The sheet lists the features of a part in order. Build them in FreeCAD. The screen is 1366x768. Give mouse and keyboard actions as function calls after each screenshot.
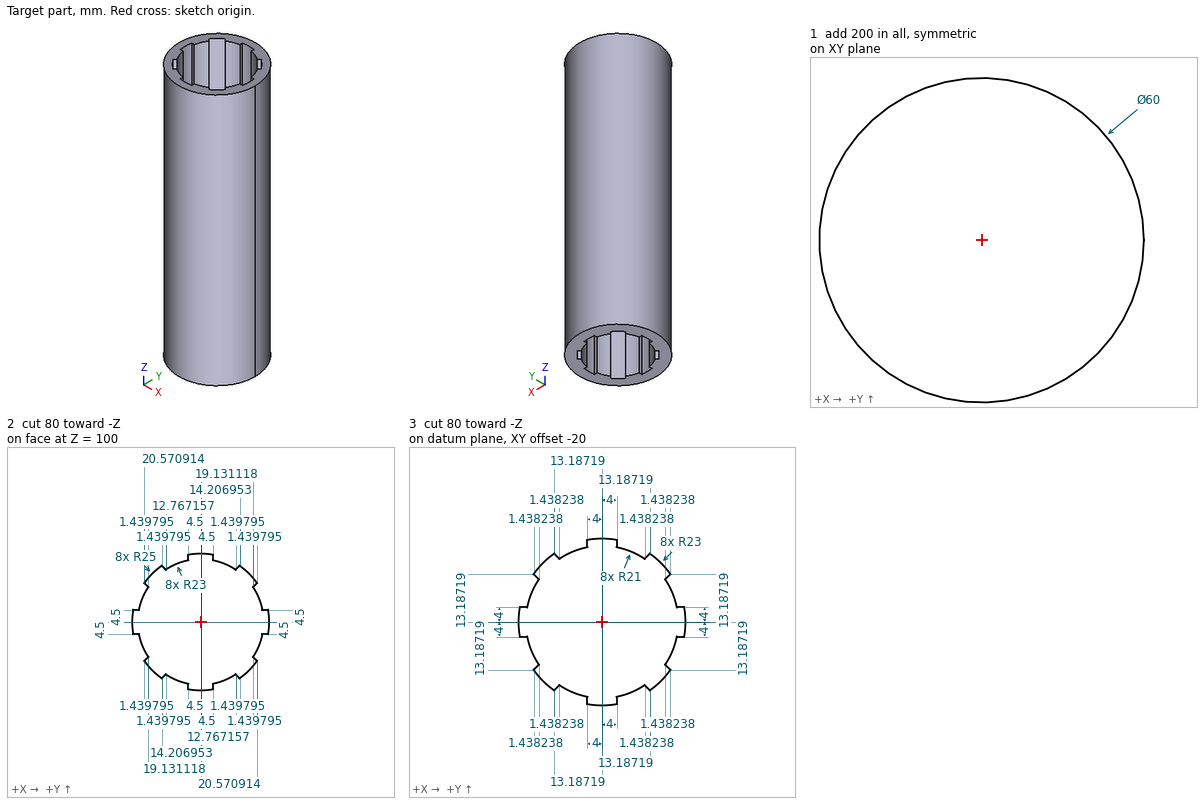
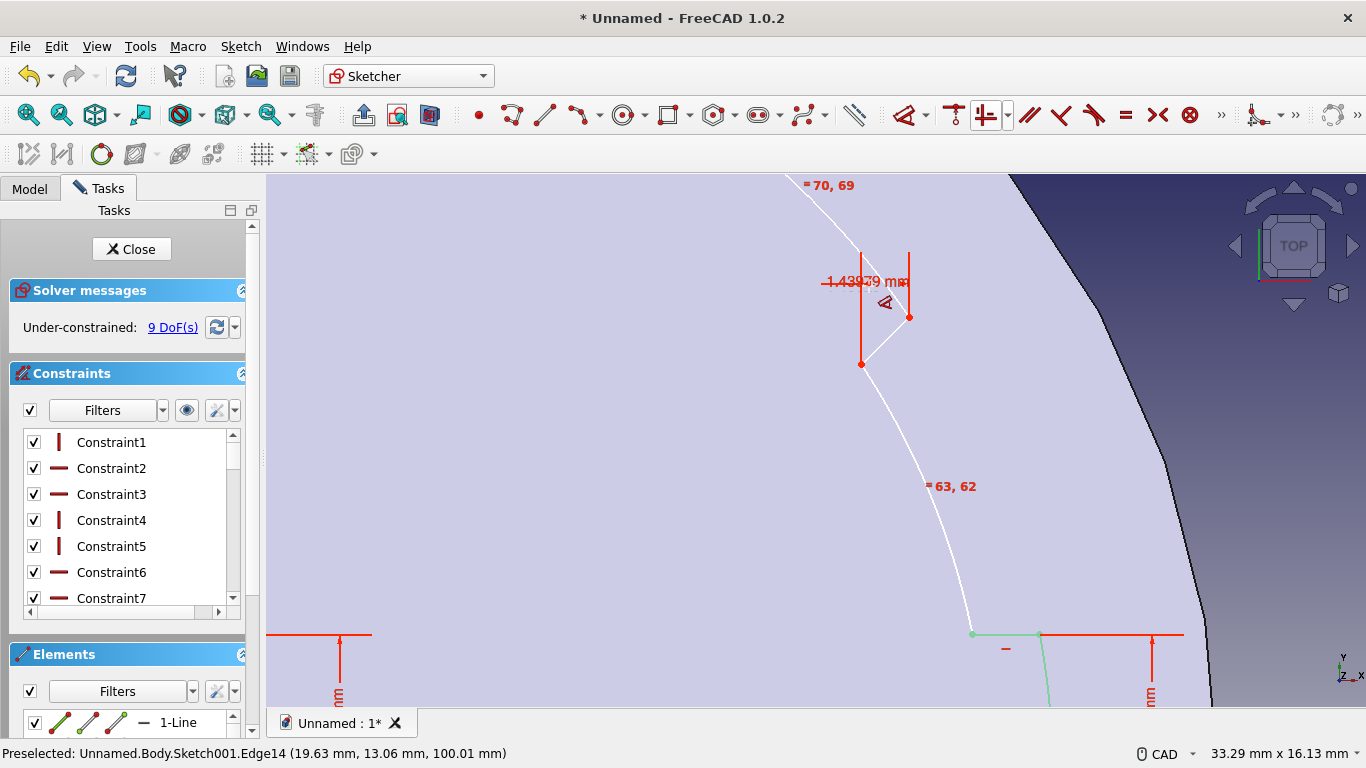
scroll(879, 354, down, 8)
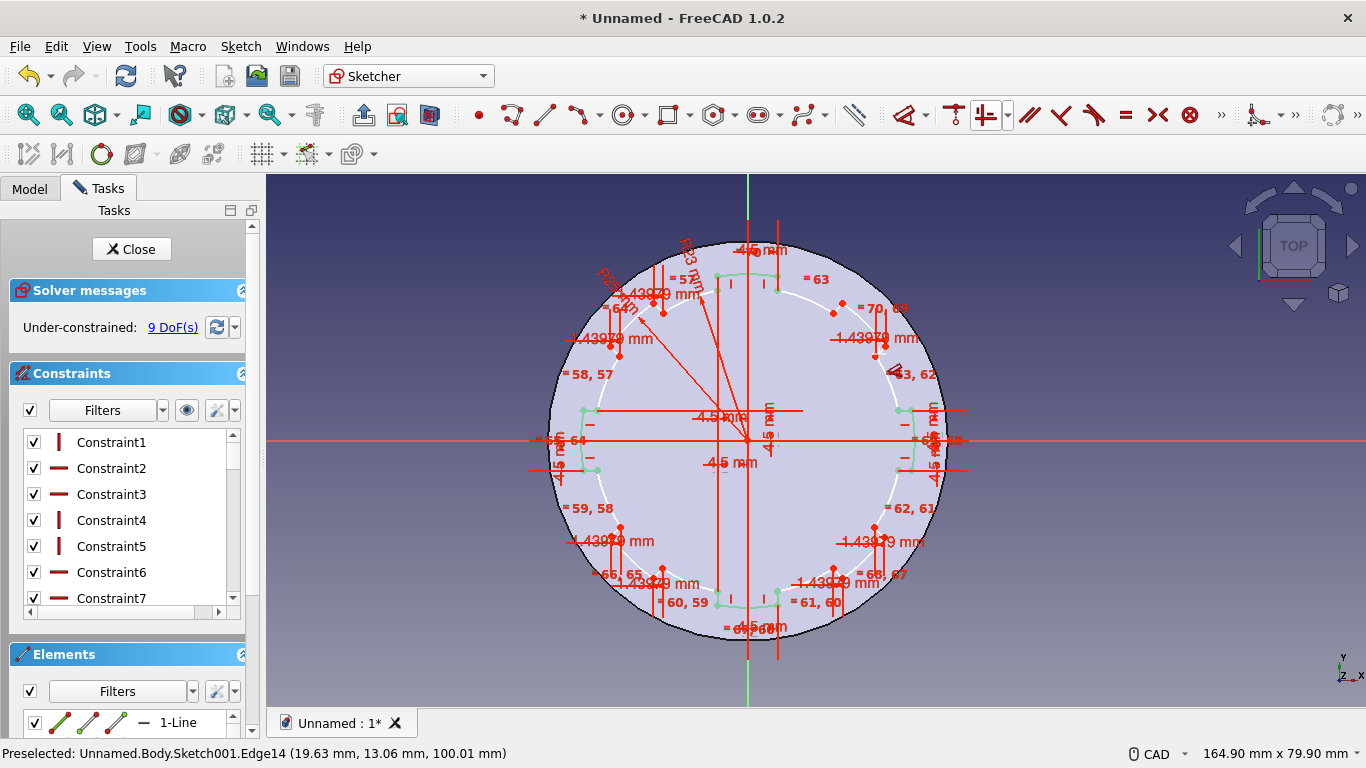
scroll(840, 307, up, 8)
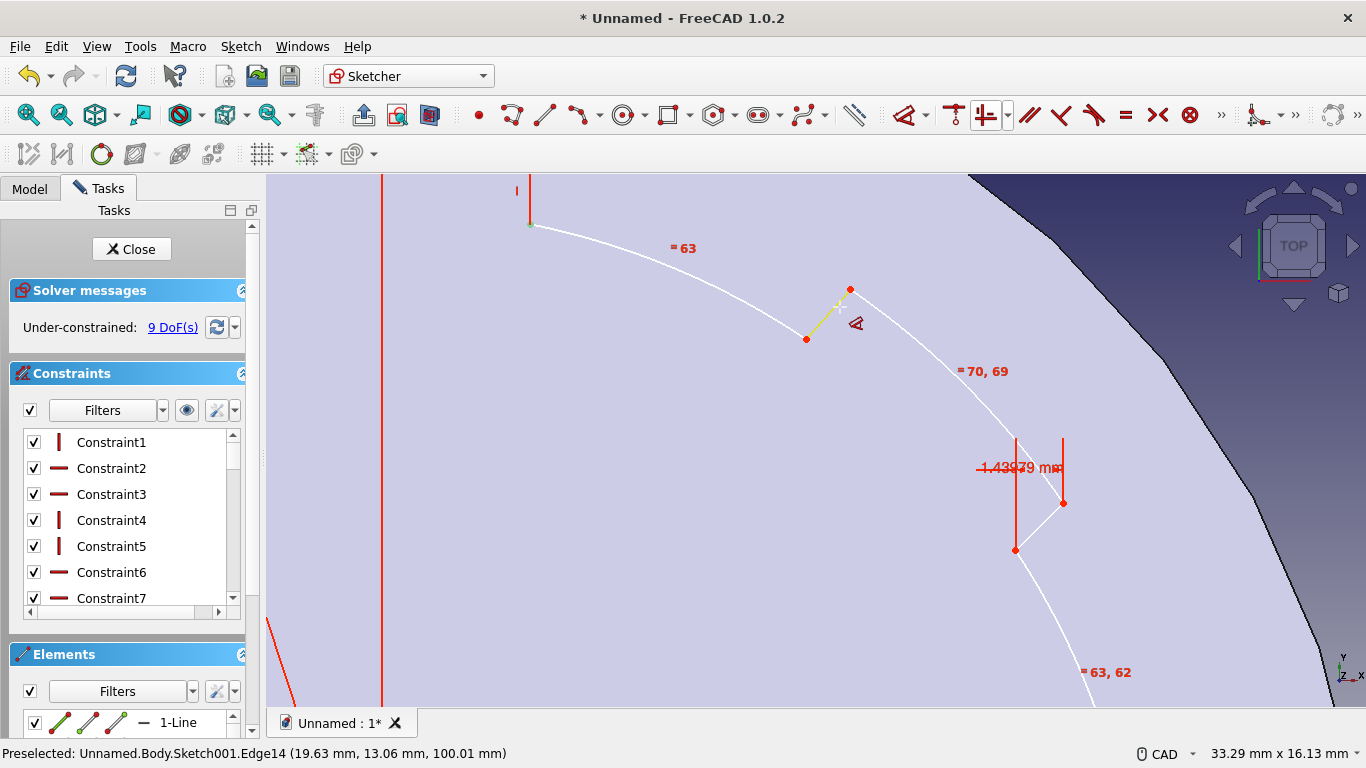
click(837, 305)
click(828, 256)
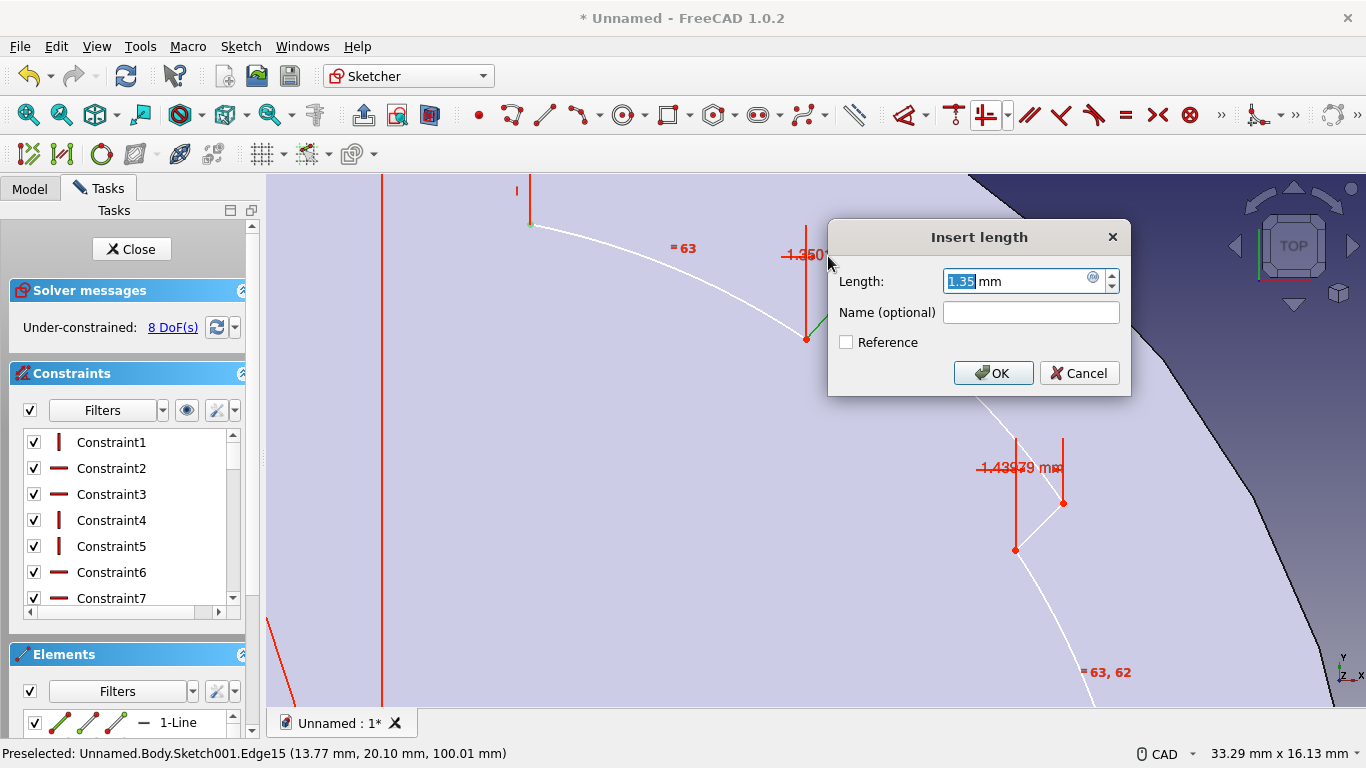
text(1.439795)
key(Return)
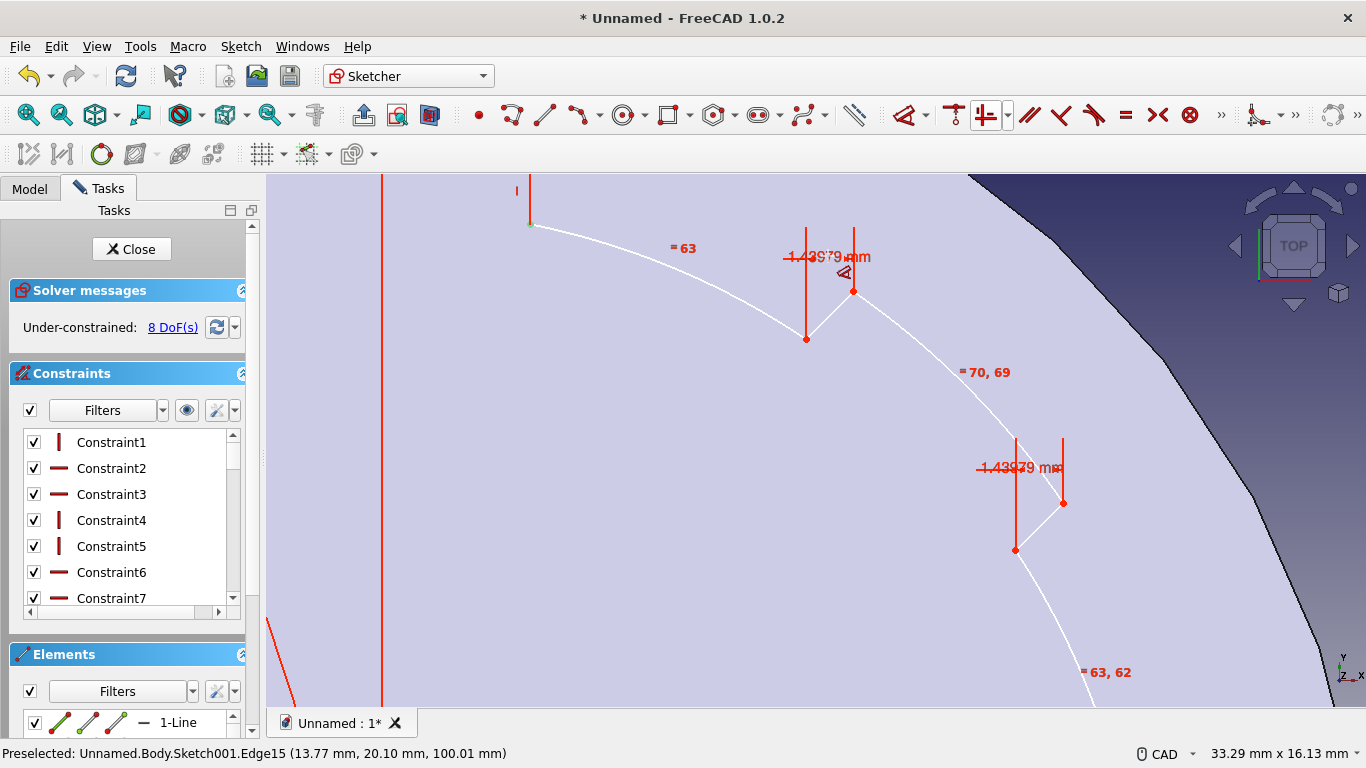
scroll(840, 307, down, 8)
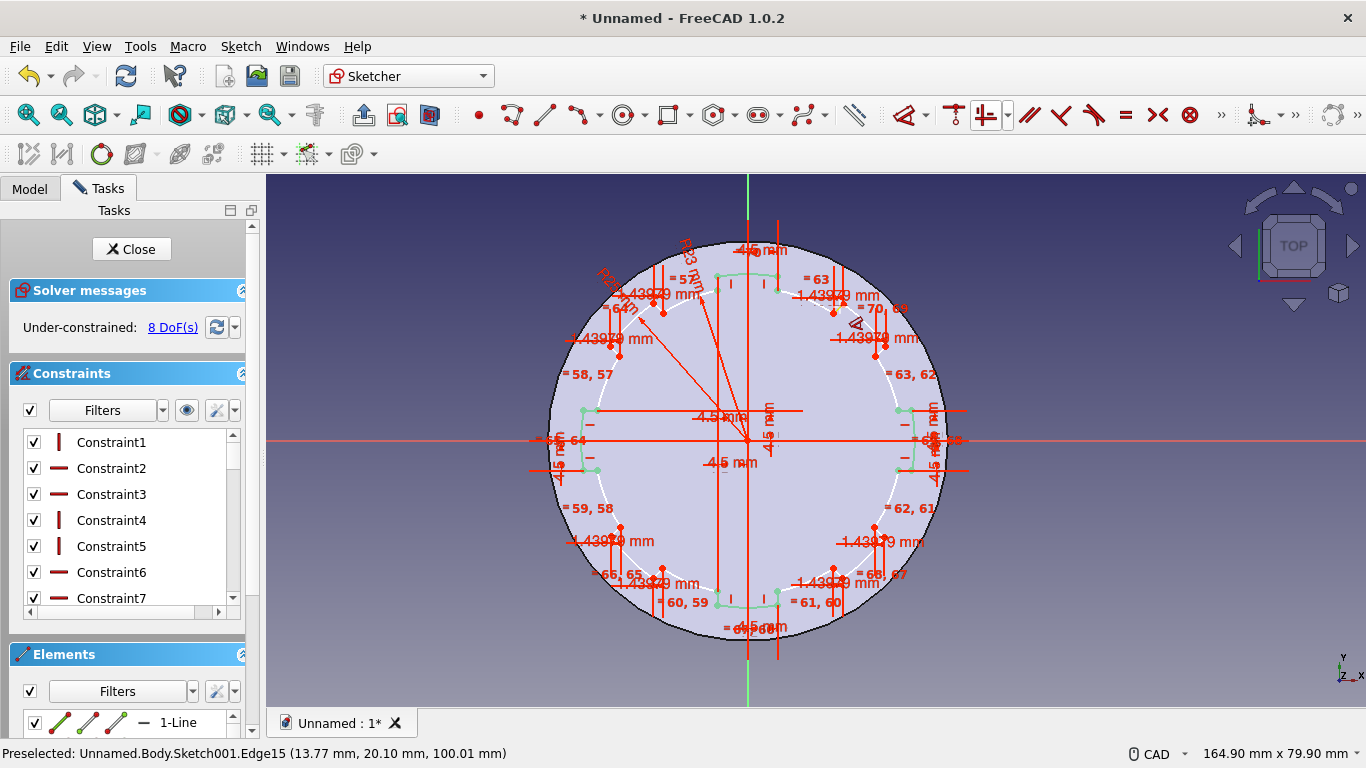
click(663, 313)
click(706, 499)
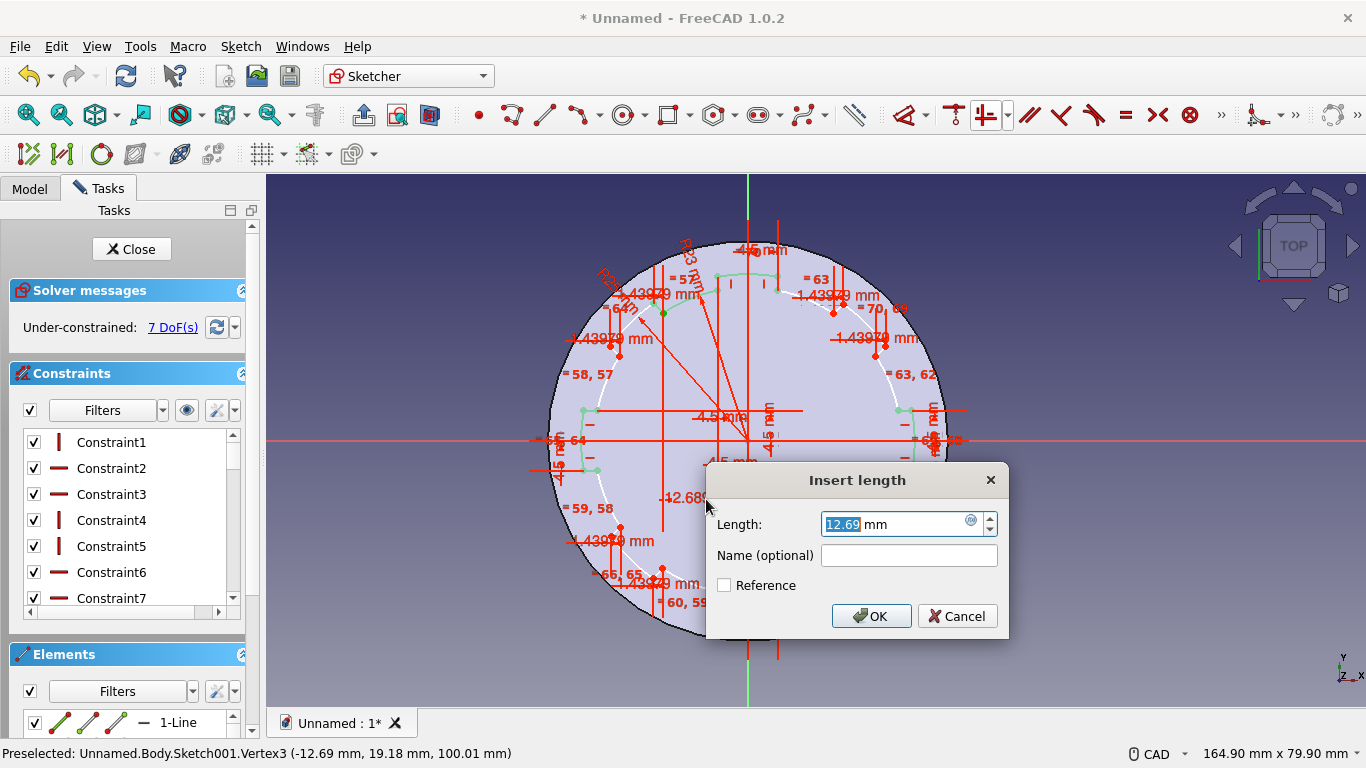
text(12.767157)
key(Return)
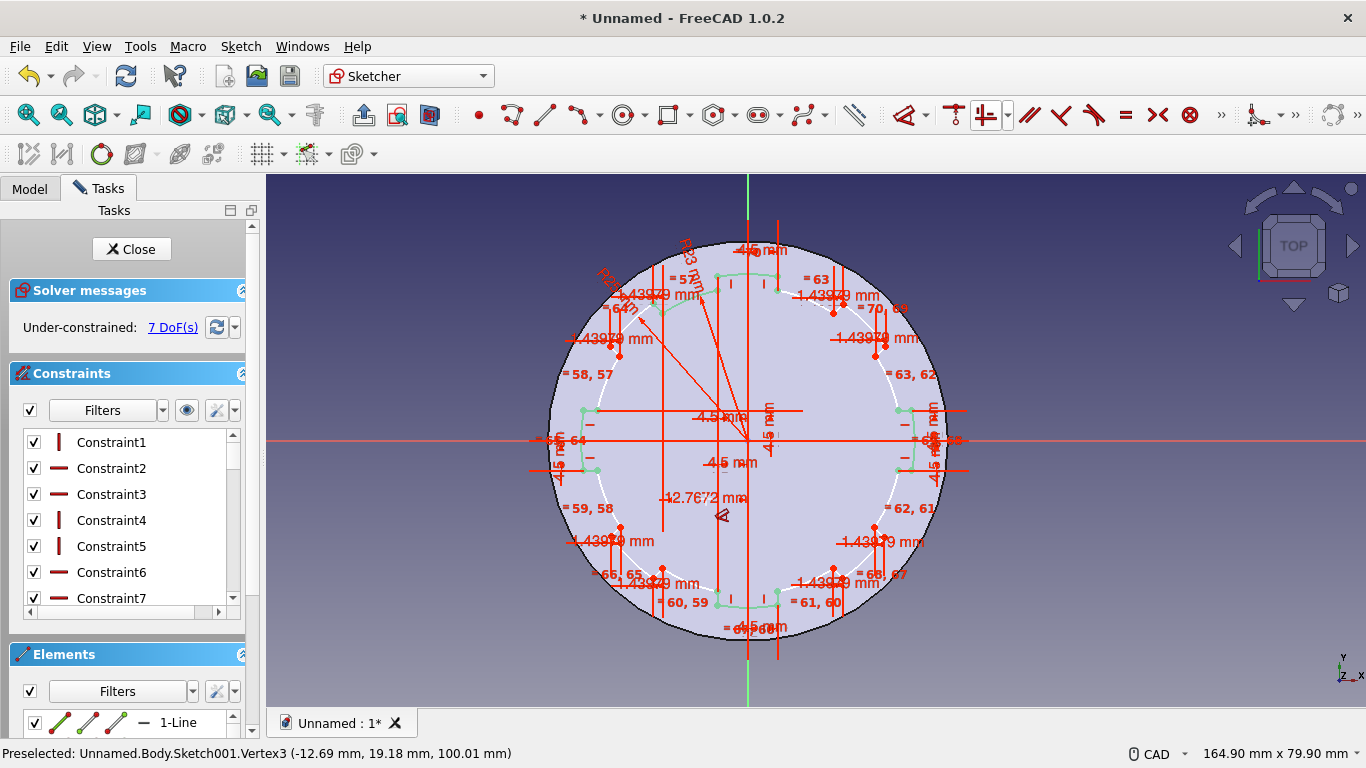
click(610, 347)
click(647, 475)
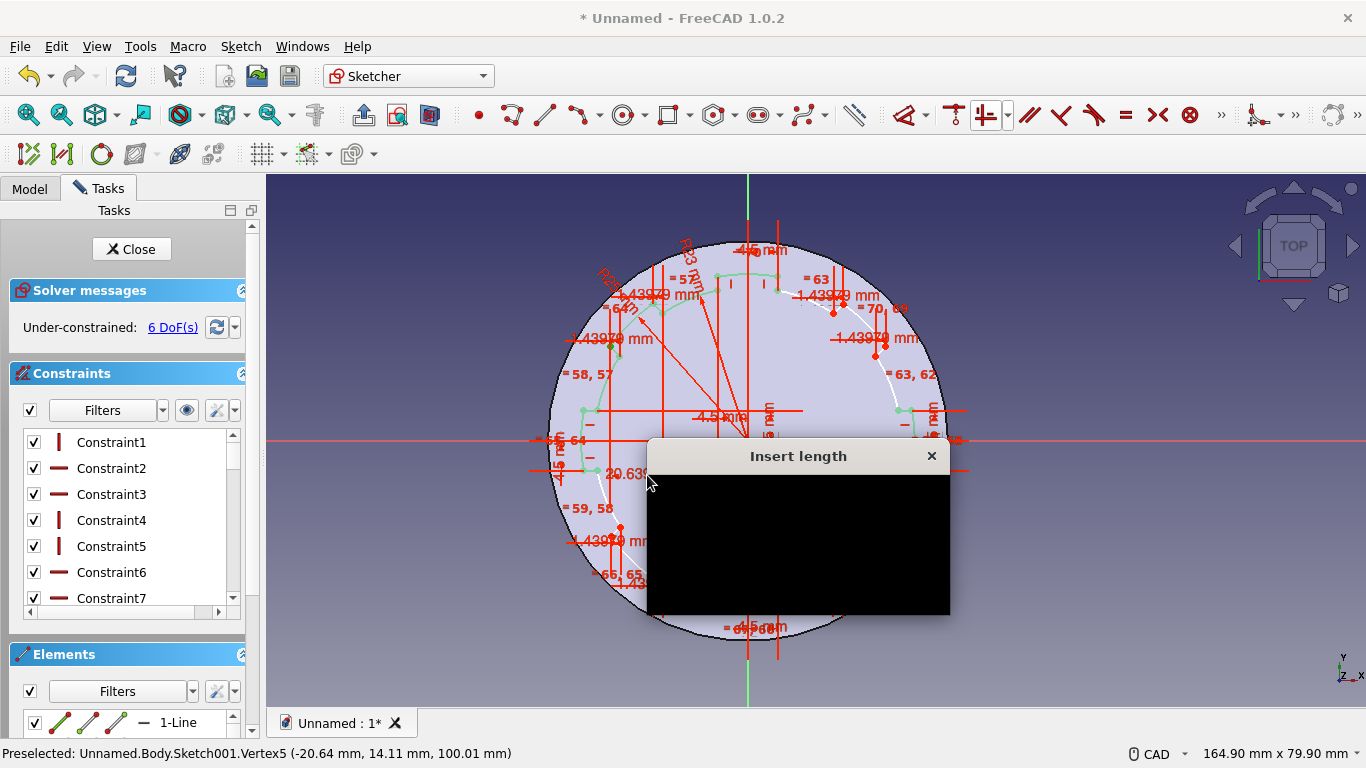
text(20.570914)
key(Return)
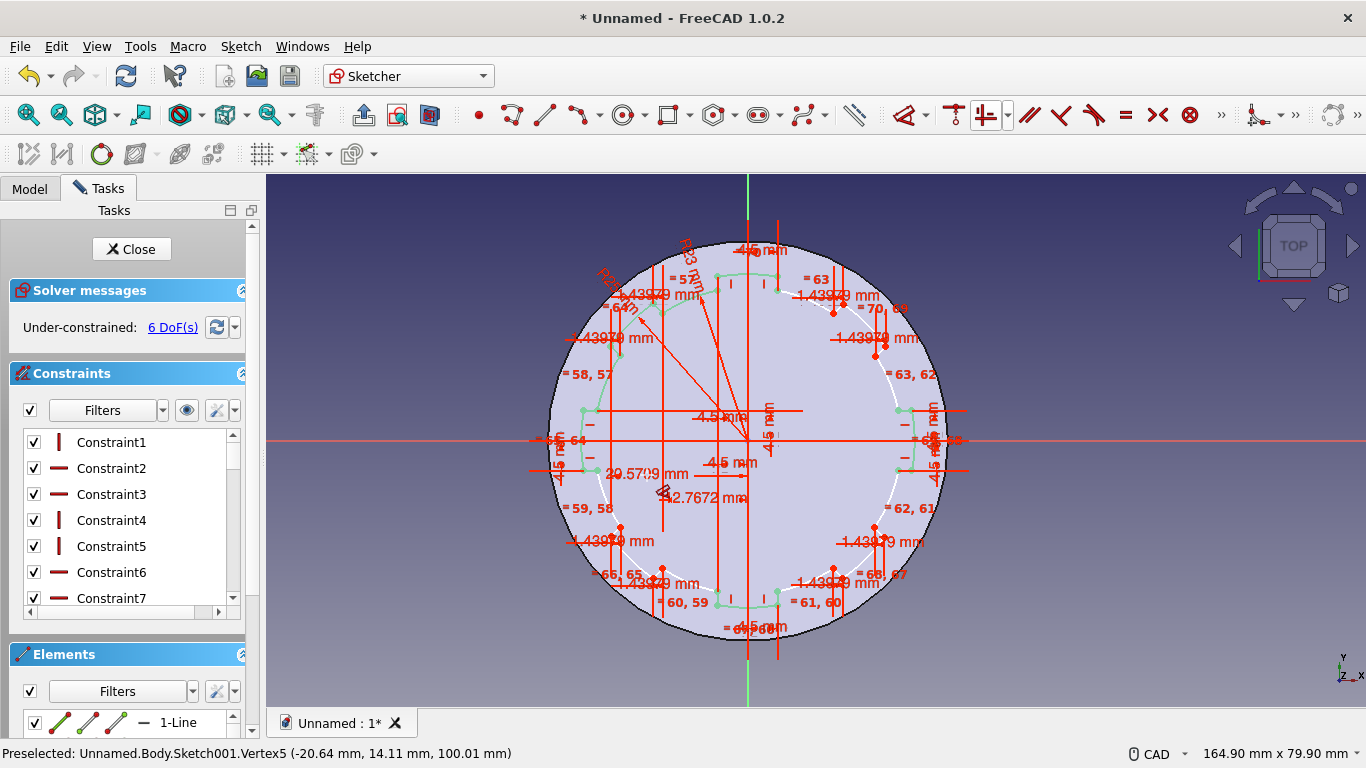
click(621, 527)
click(684, 561)